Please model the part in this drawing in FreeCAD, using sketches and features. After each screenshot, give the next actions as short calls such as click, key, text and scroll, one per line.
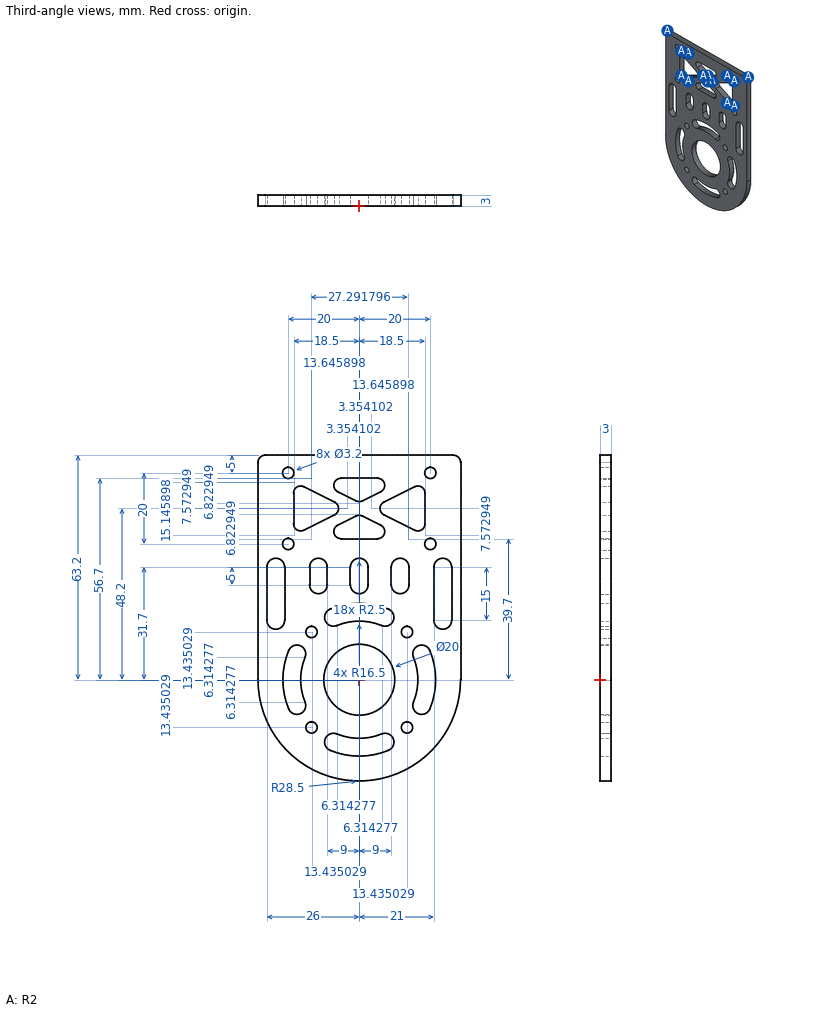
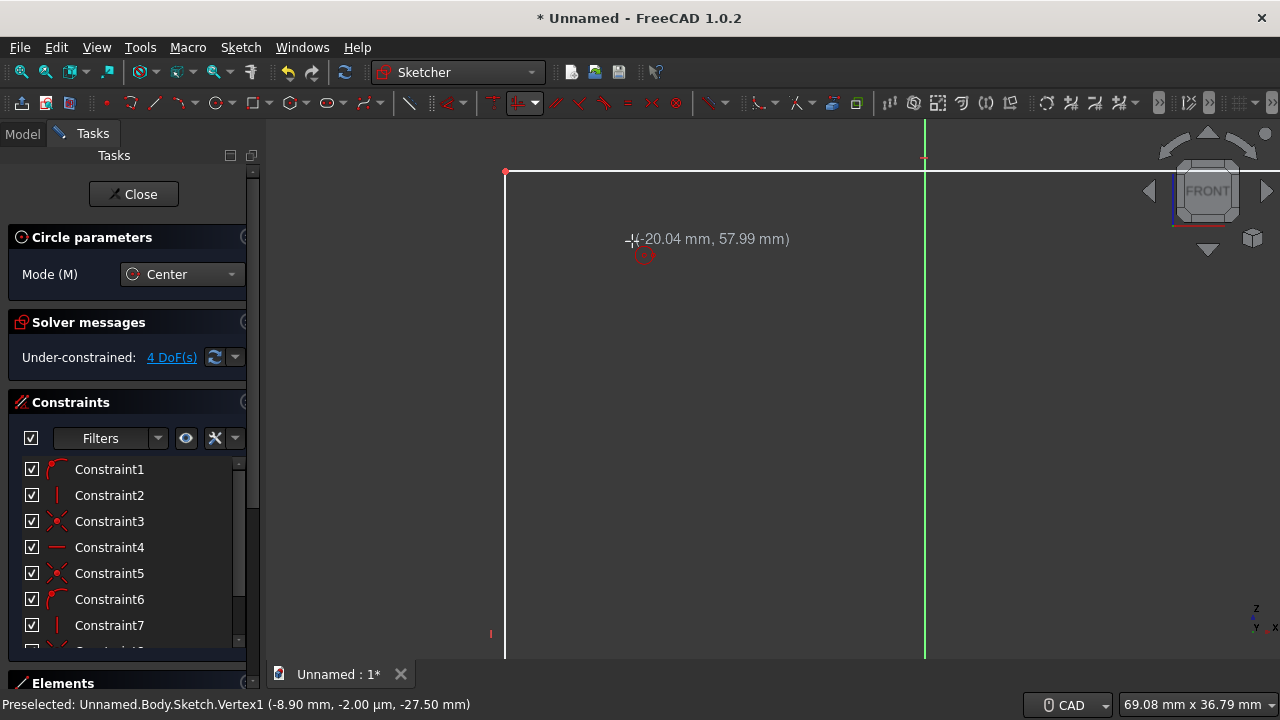
scroll(632, 241, down, 7)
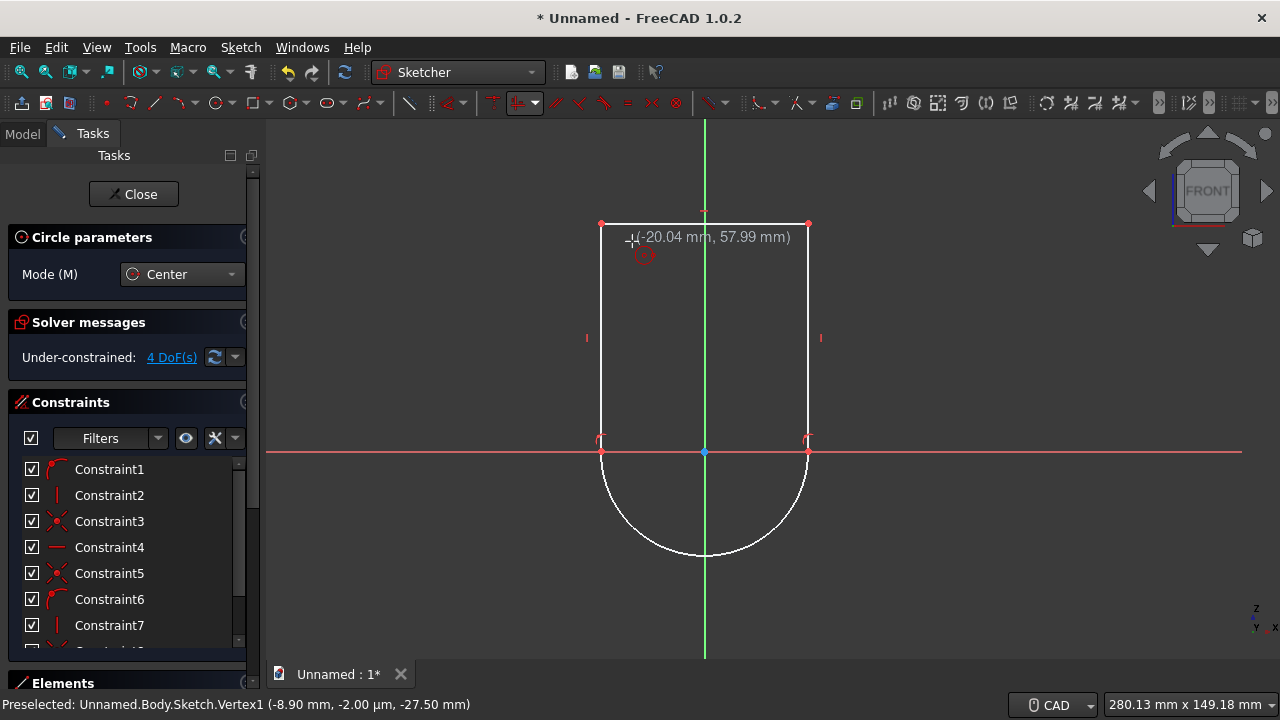
click(632, 241)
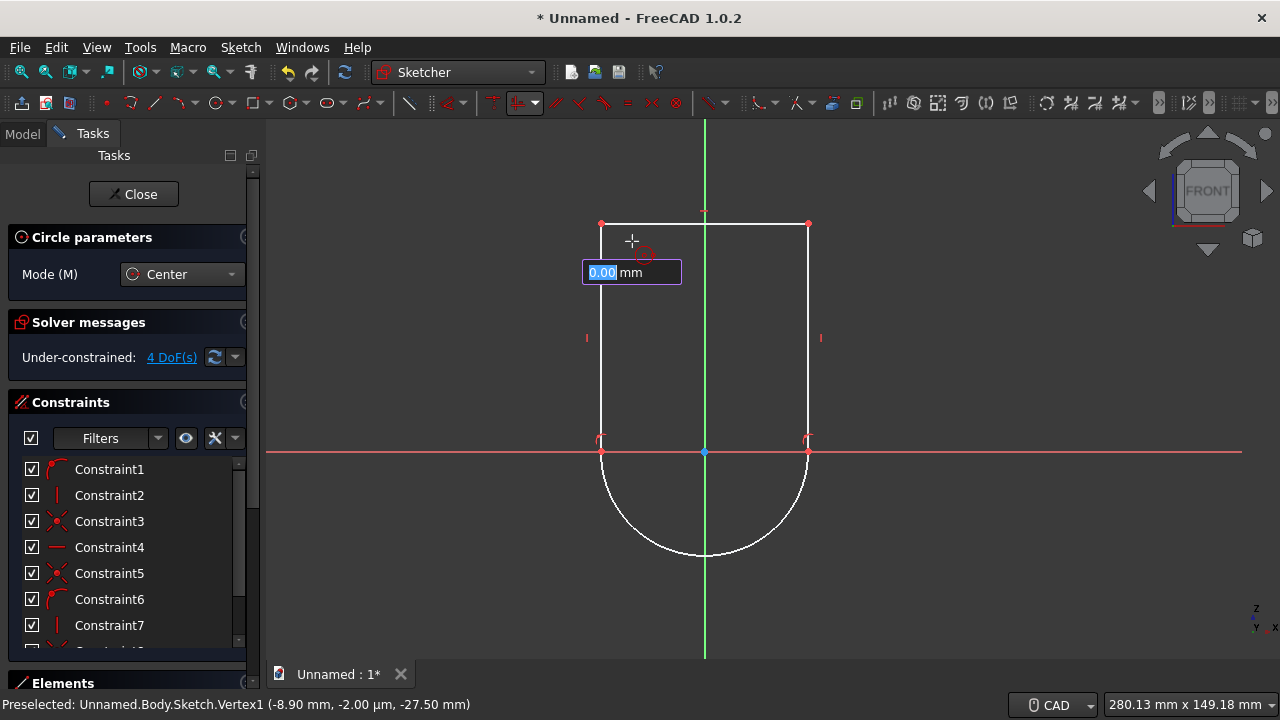
scroll(636, 237, up, 6)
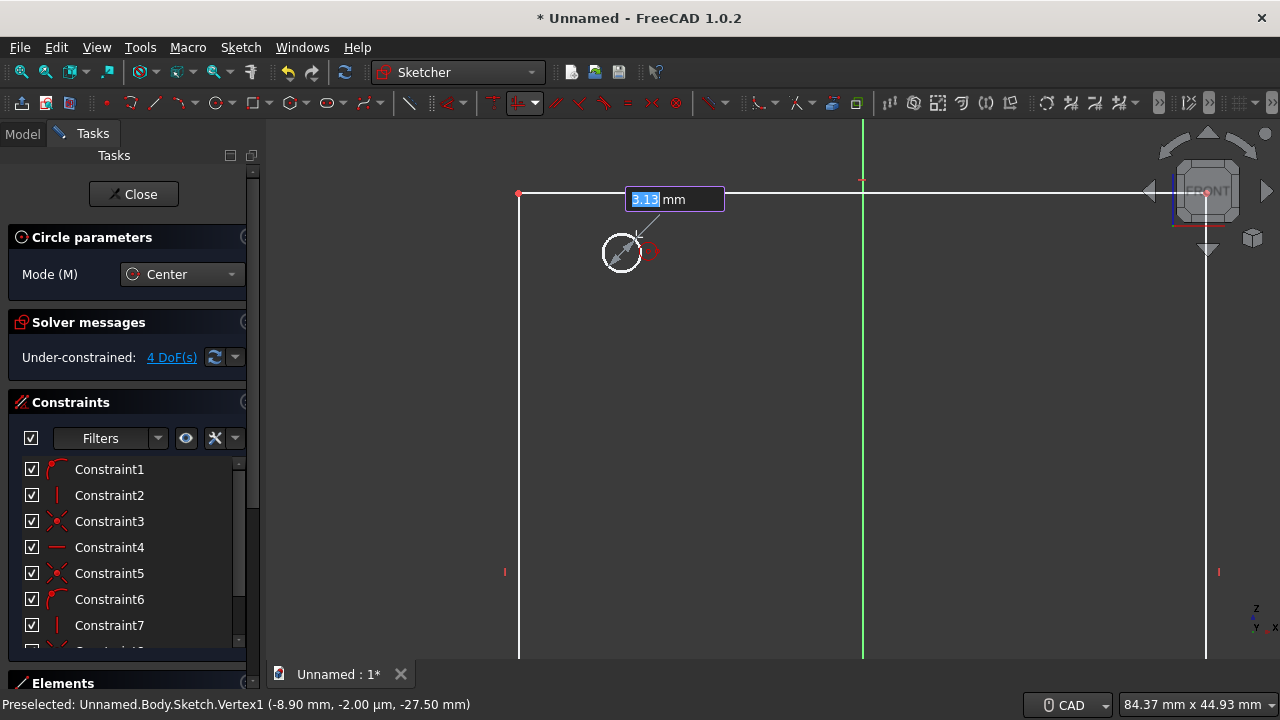
click(636, 237)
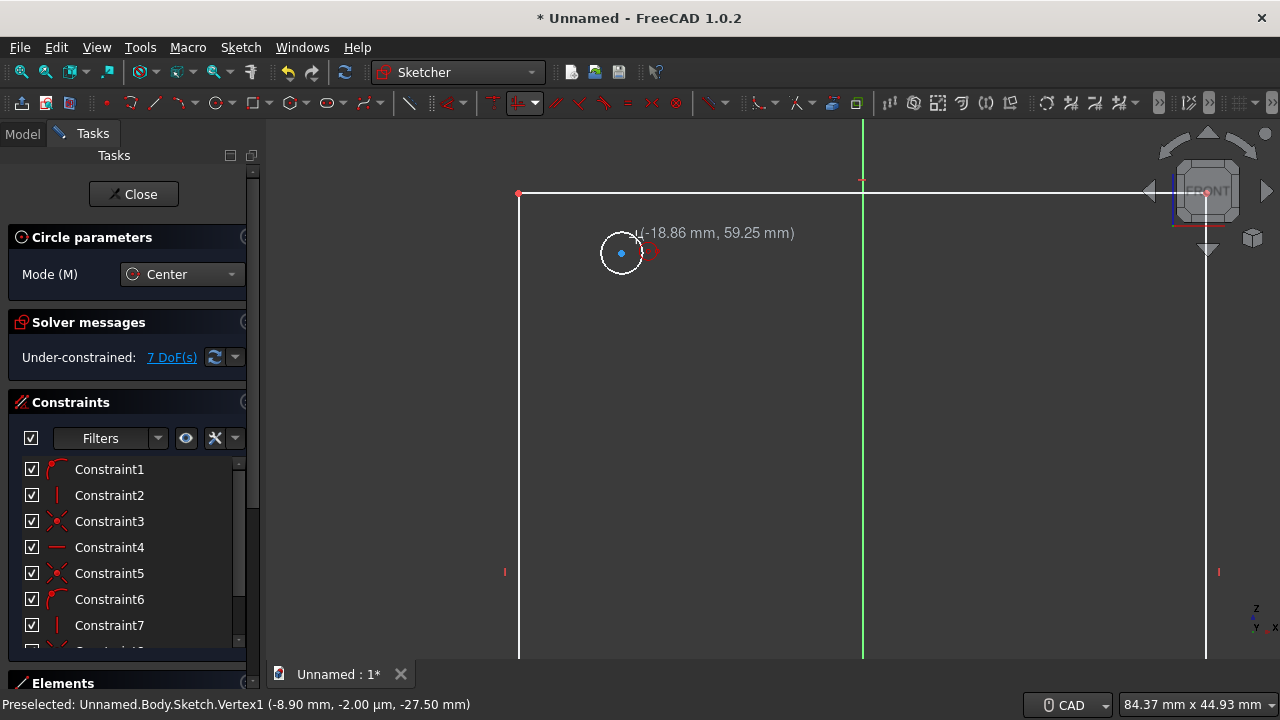
click(622, 491)
click(636, 477)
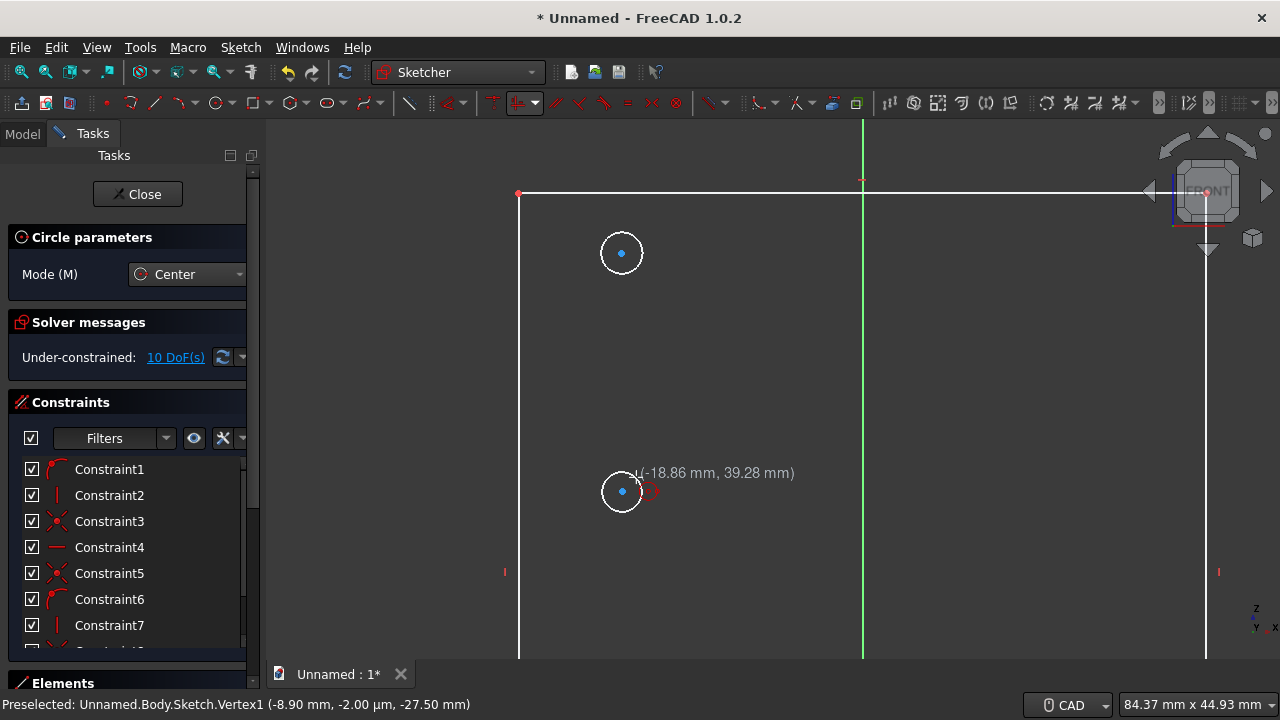
click(1103, 251)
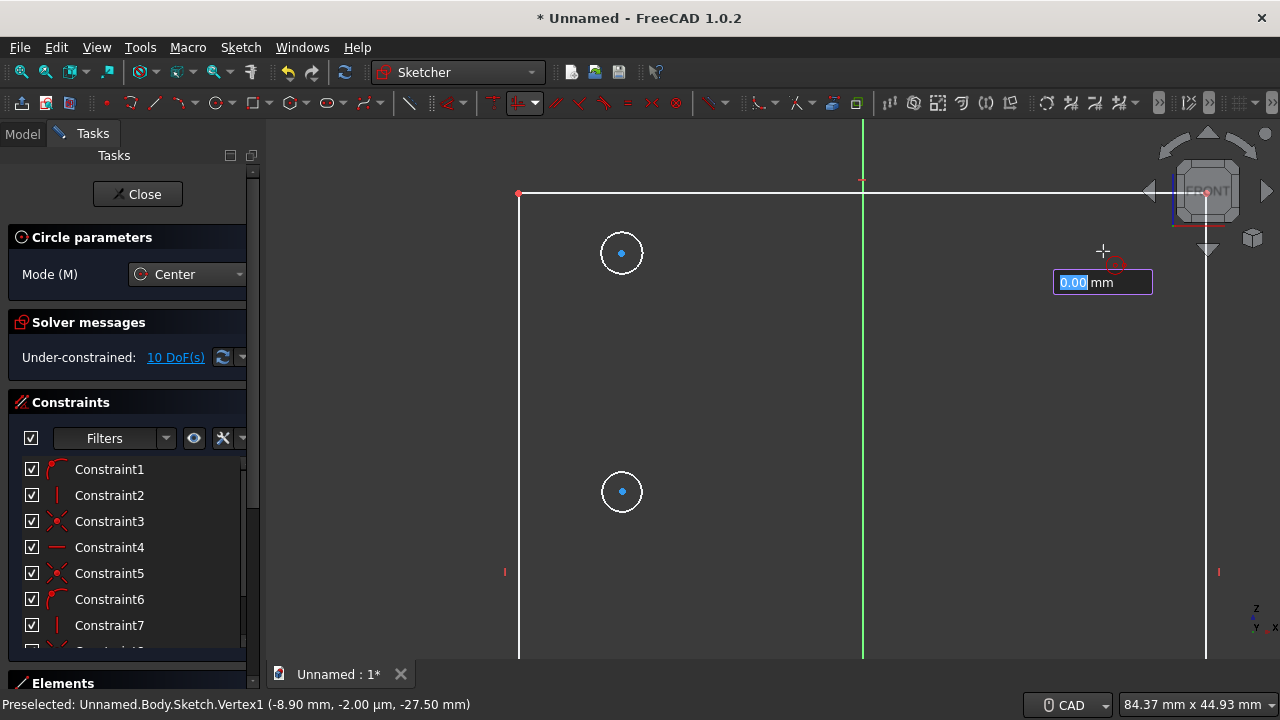
scroll(636, 237, down, 6)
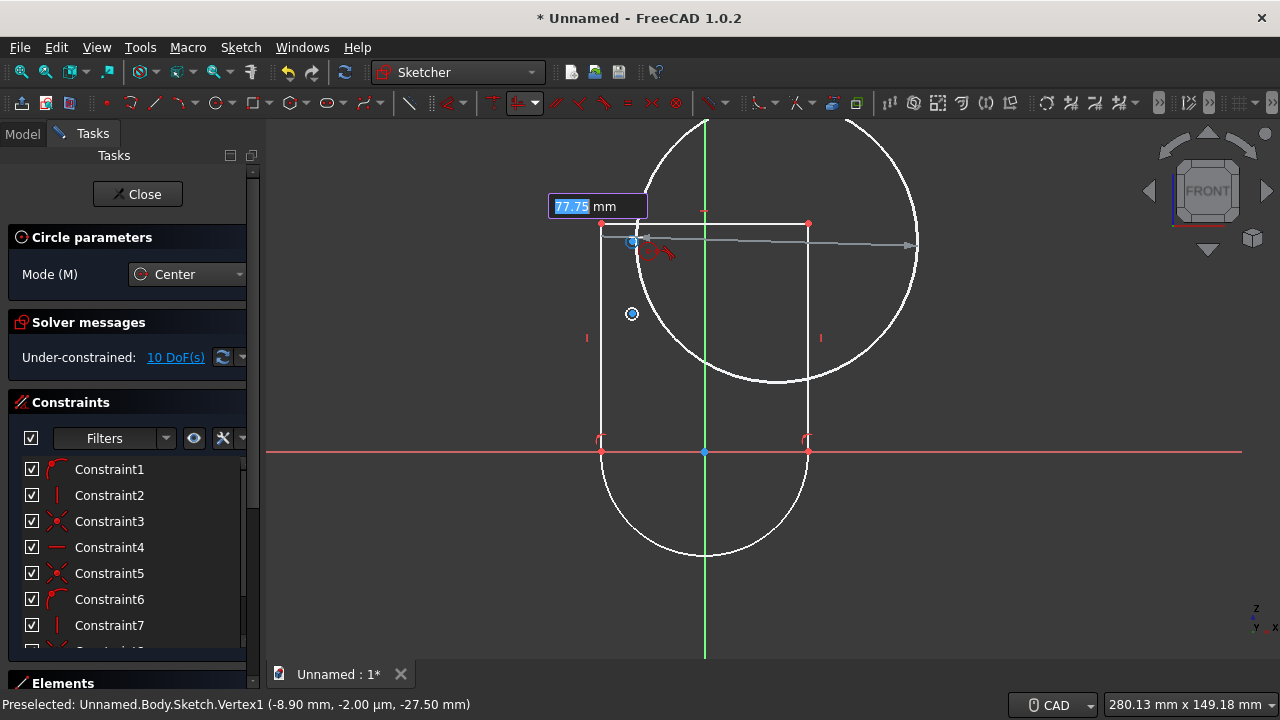
scroll(781, 237, up, 6)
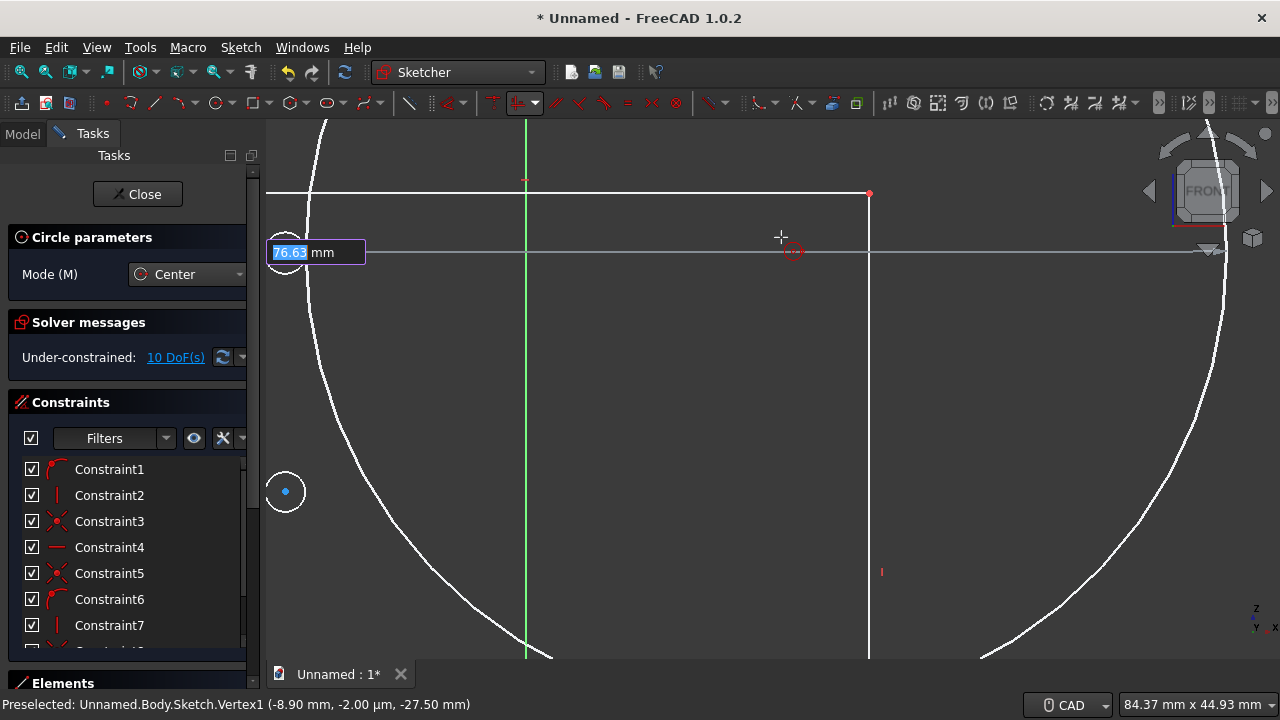
click(780, 237)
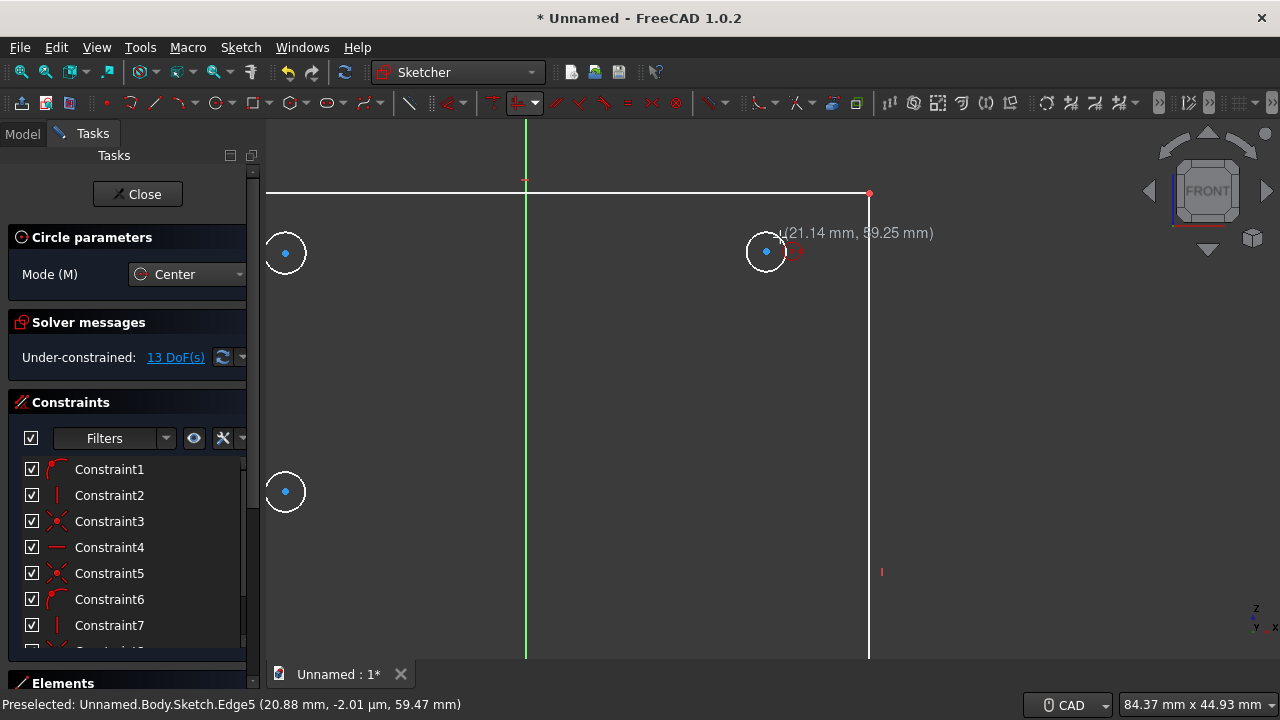
click(766, 491)
click(780, 477)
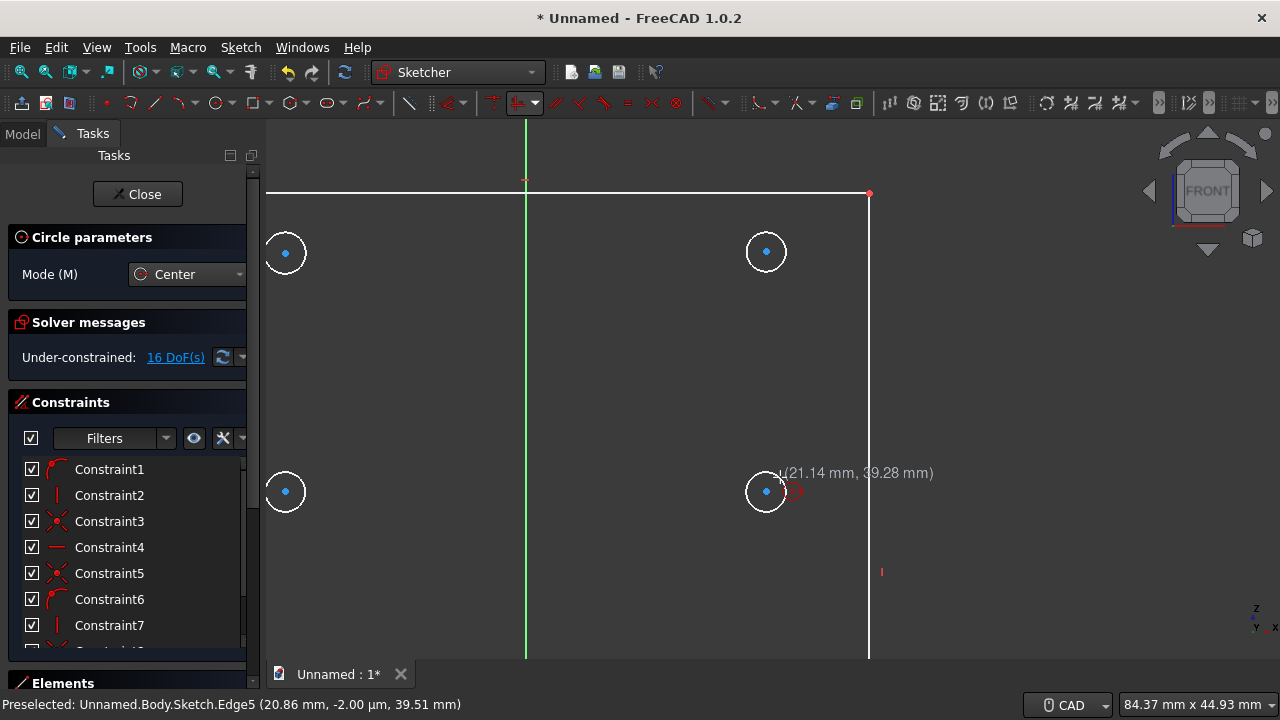
scroll(781, 237, down, 6)